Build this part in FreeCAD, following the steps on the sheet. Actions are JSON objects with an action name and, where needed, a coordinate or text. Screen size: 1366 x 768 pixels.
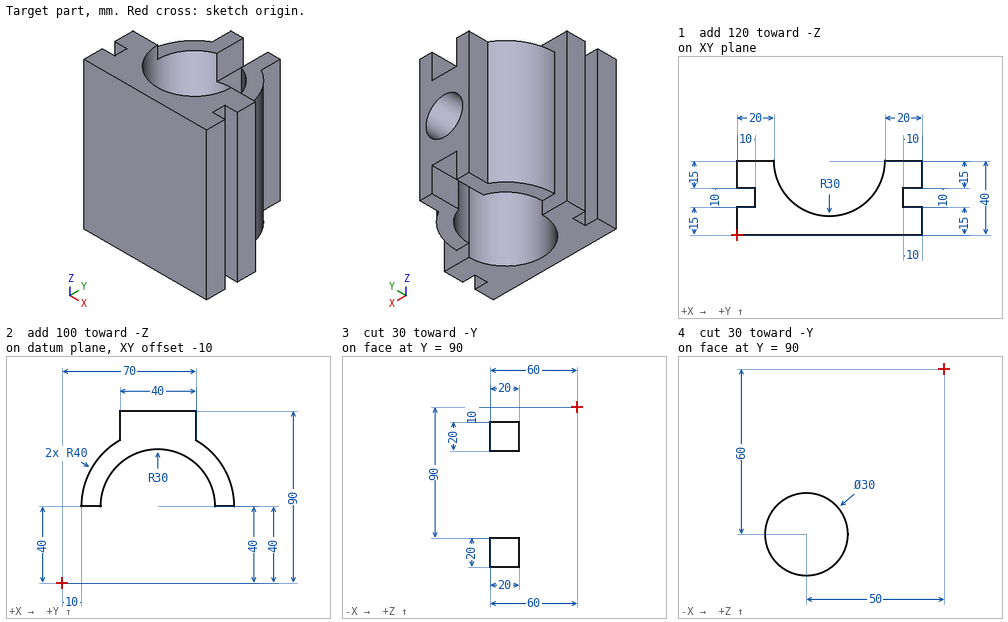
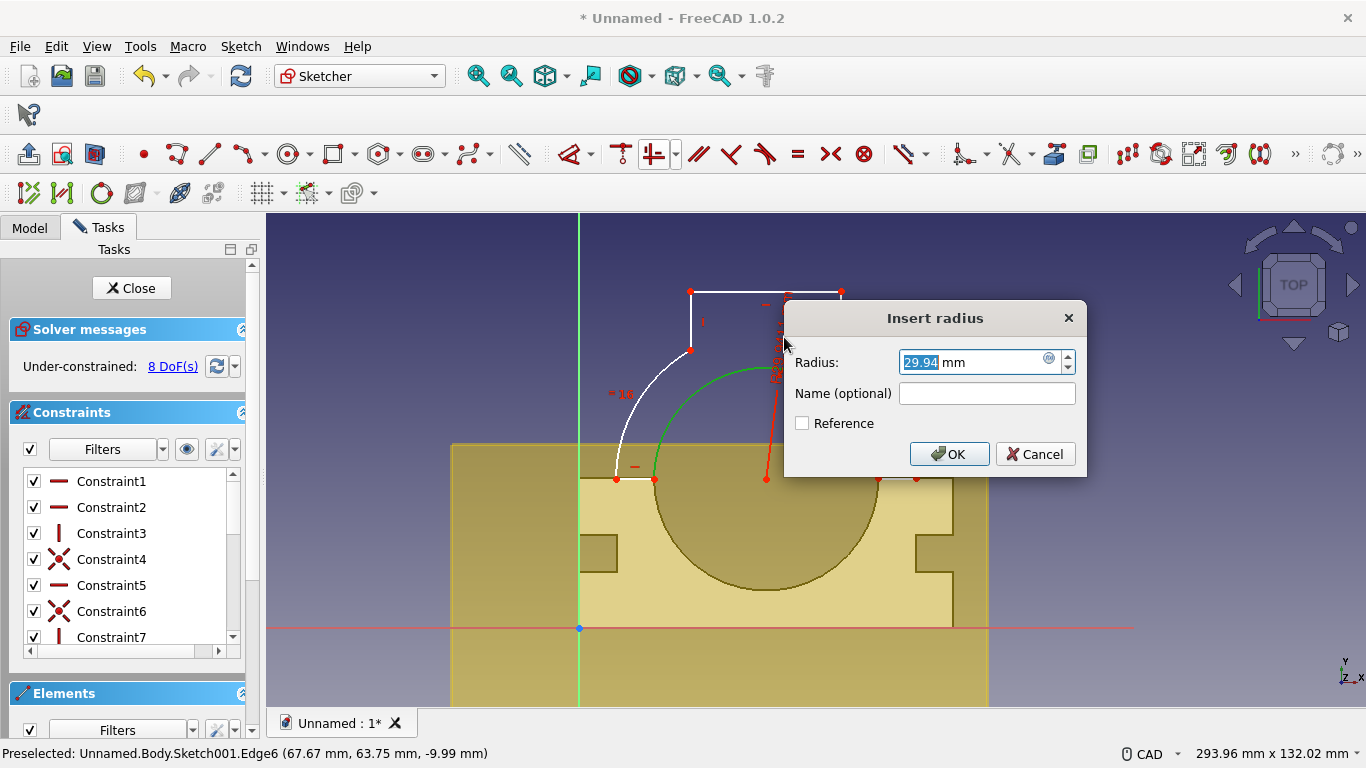
{"action": "type", "text": "30"}
{"action": "key", "text": "Return"}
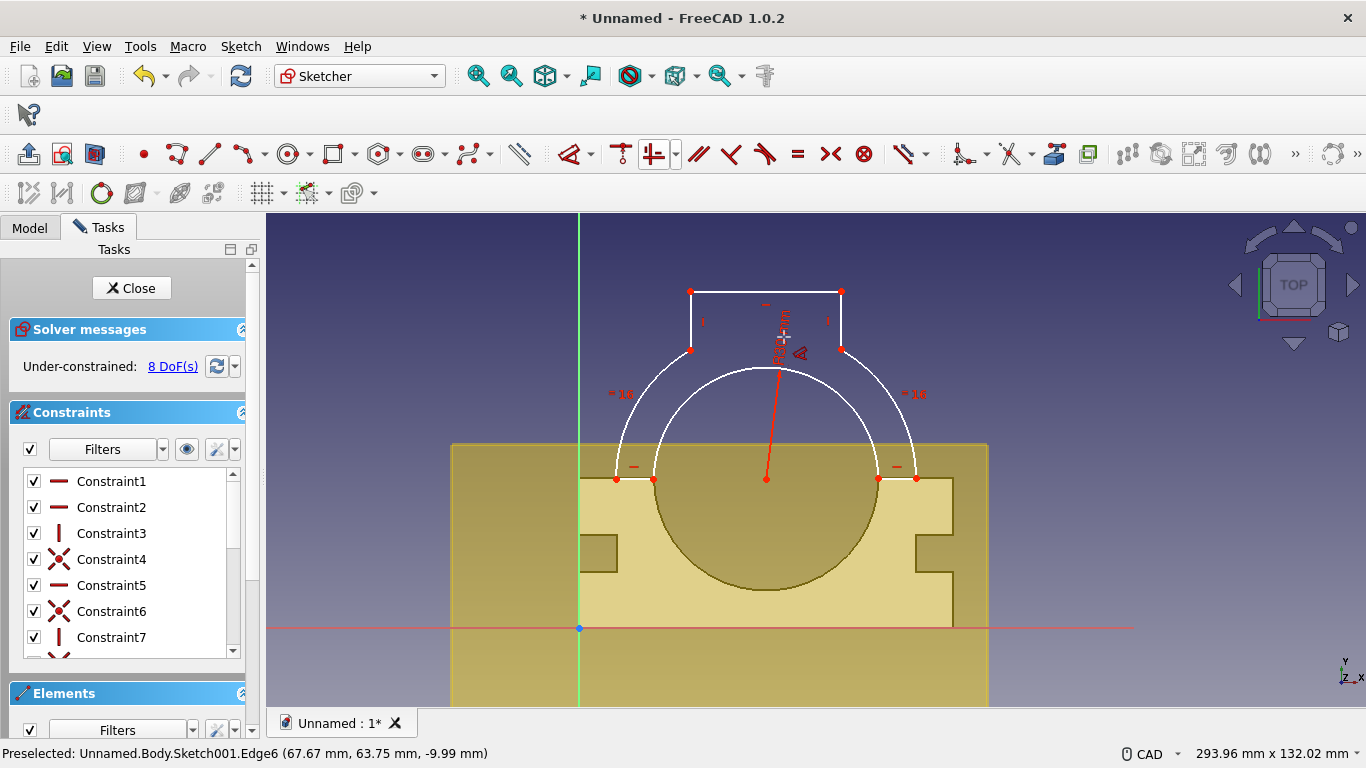
{"action": "left_click", "coordinate": [909, 433]}
{"action": "left_click", "coordinate": [939, 423]}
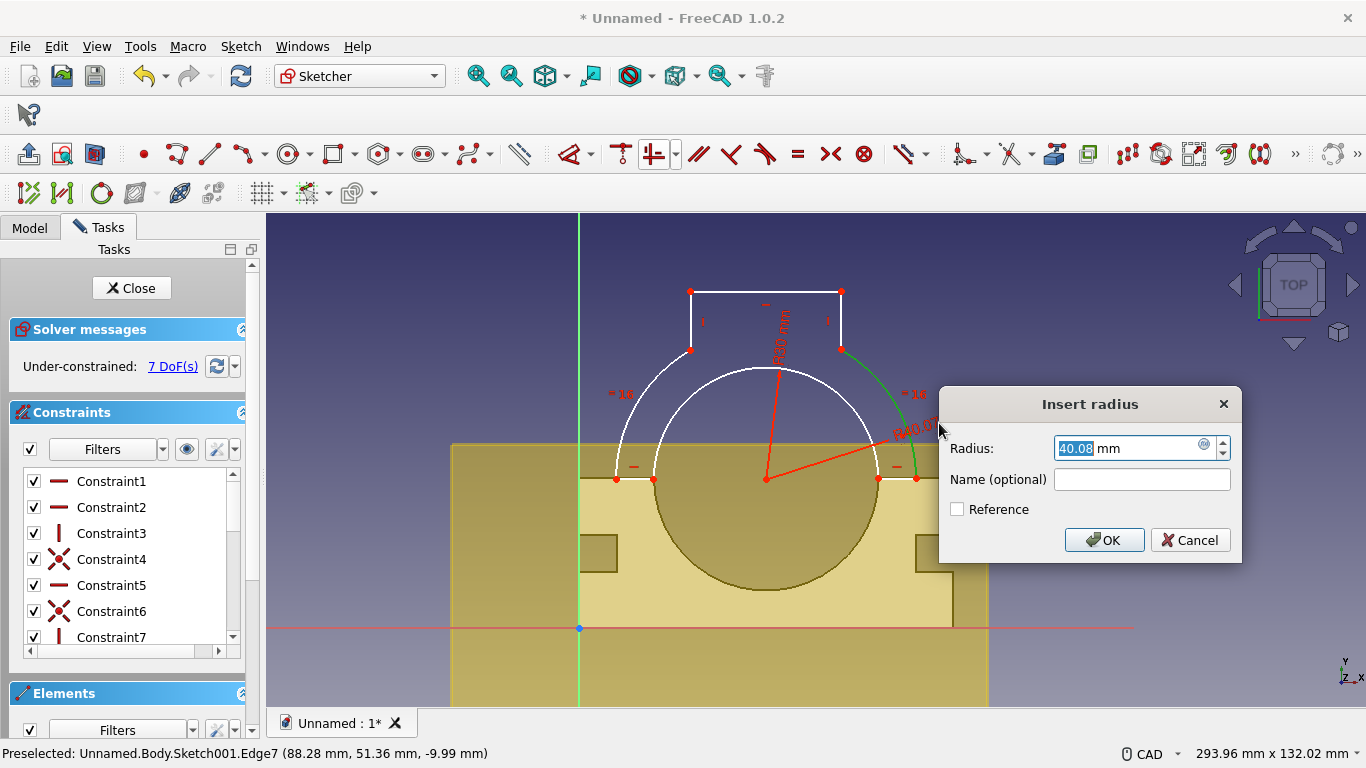
{"action": "type", "text": "40"}
{"action": "key", "text": "Return"}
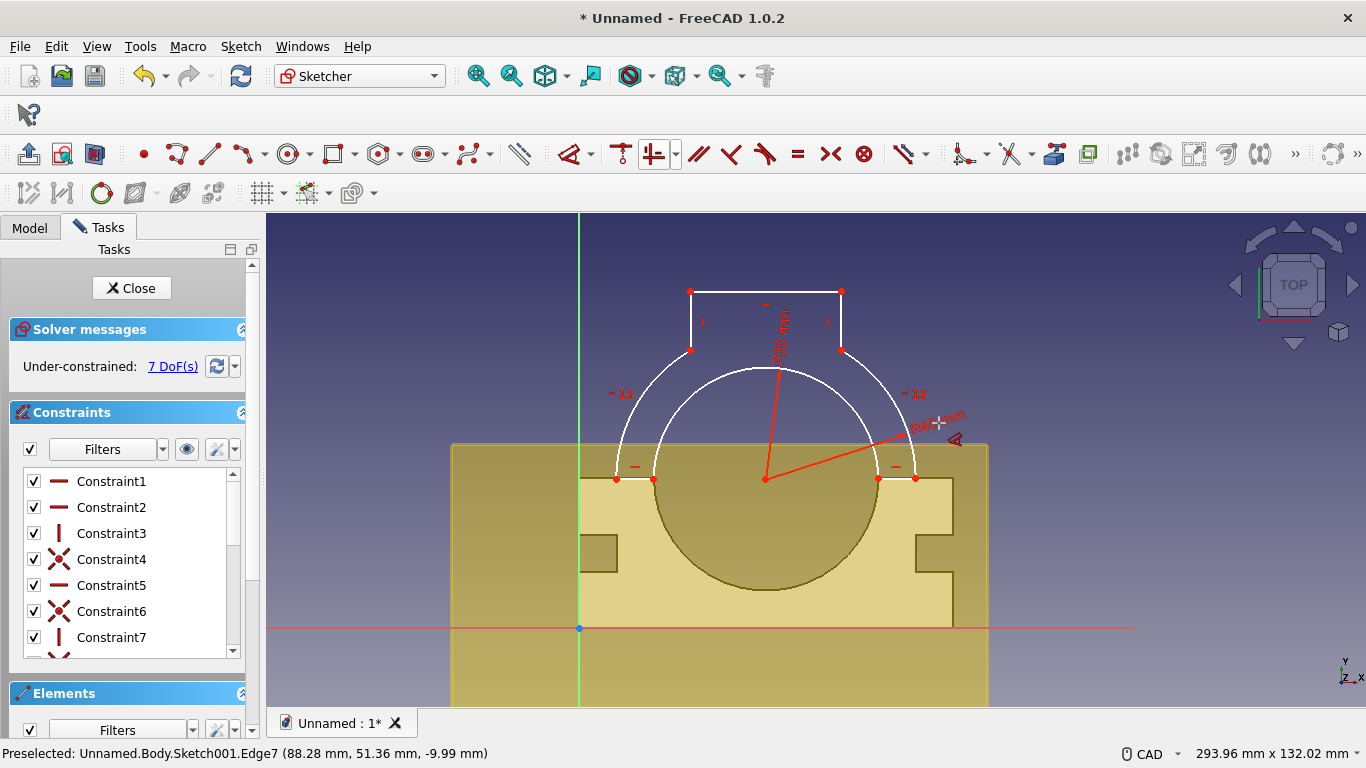
{"action": "left_click", "coordinate": [796, 292]}
{"action": "left_click", "coordinate": [766, 258]}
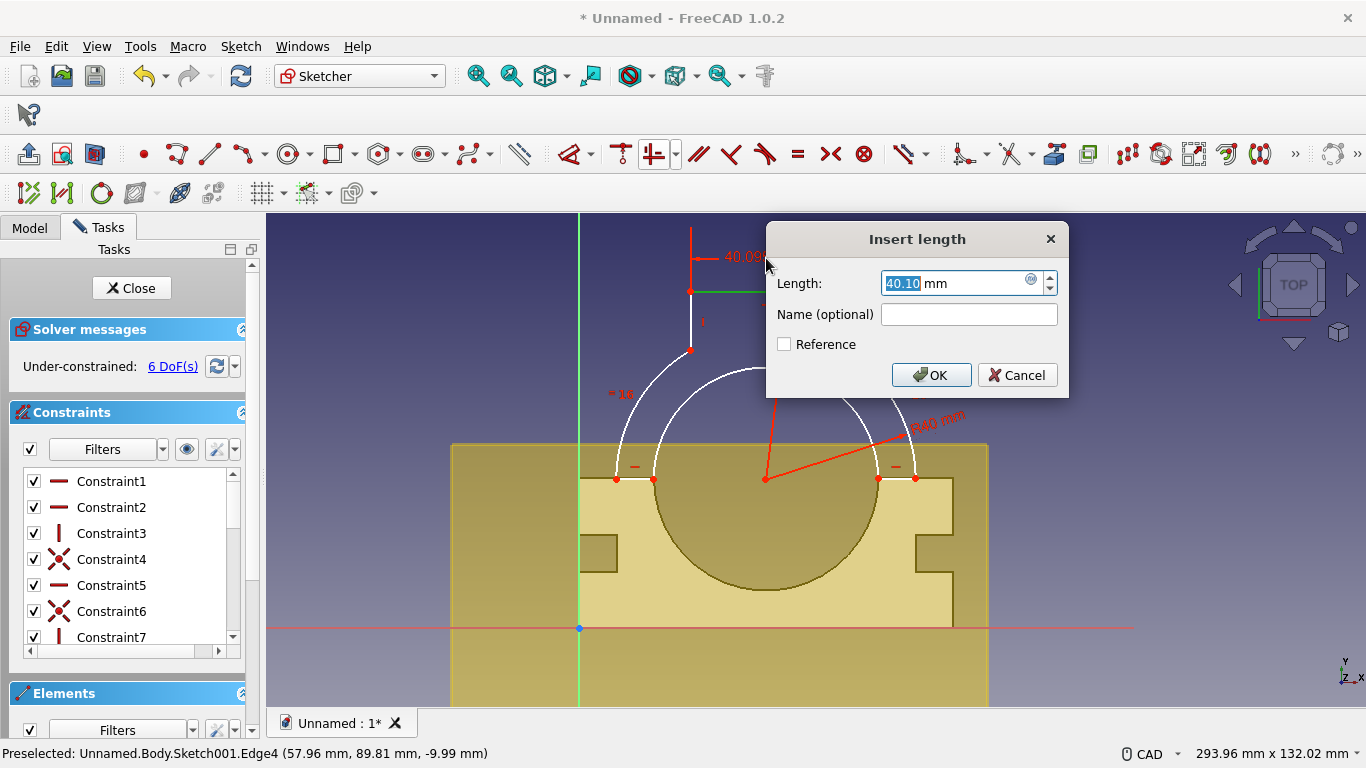
{"action": "type", "text": "40"}
{"action": "key", "text": "Return"}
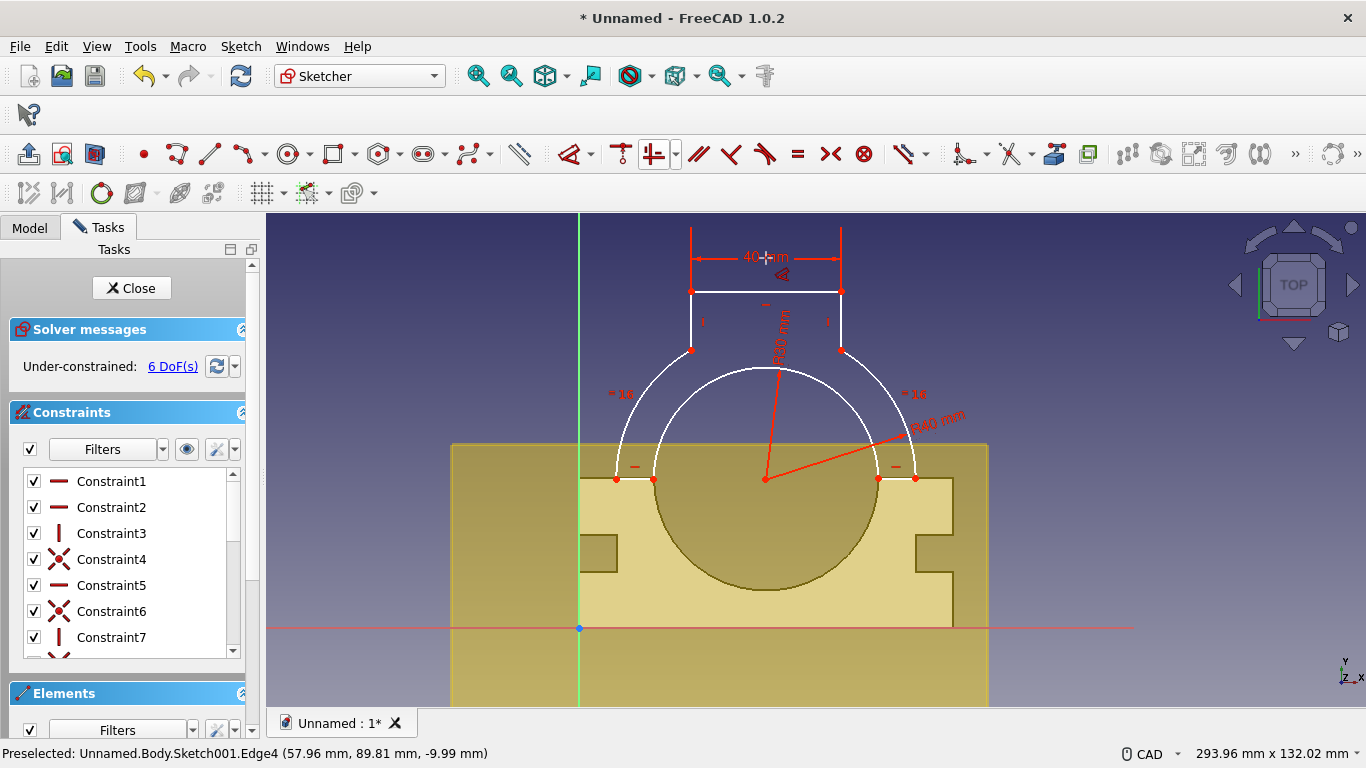
{"action": "left_click", "coordinate": [616, 479]}
{"action": "left_click", "coordinate": [598, 662]}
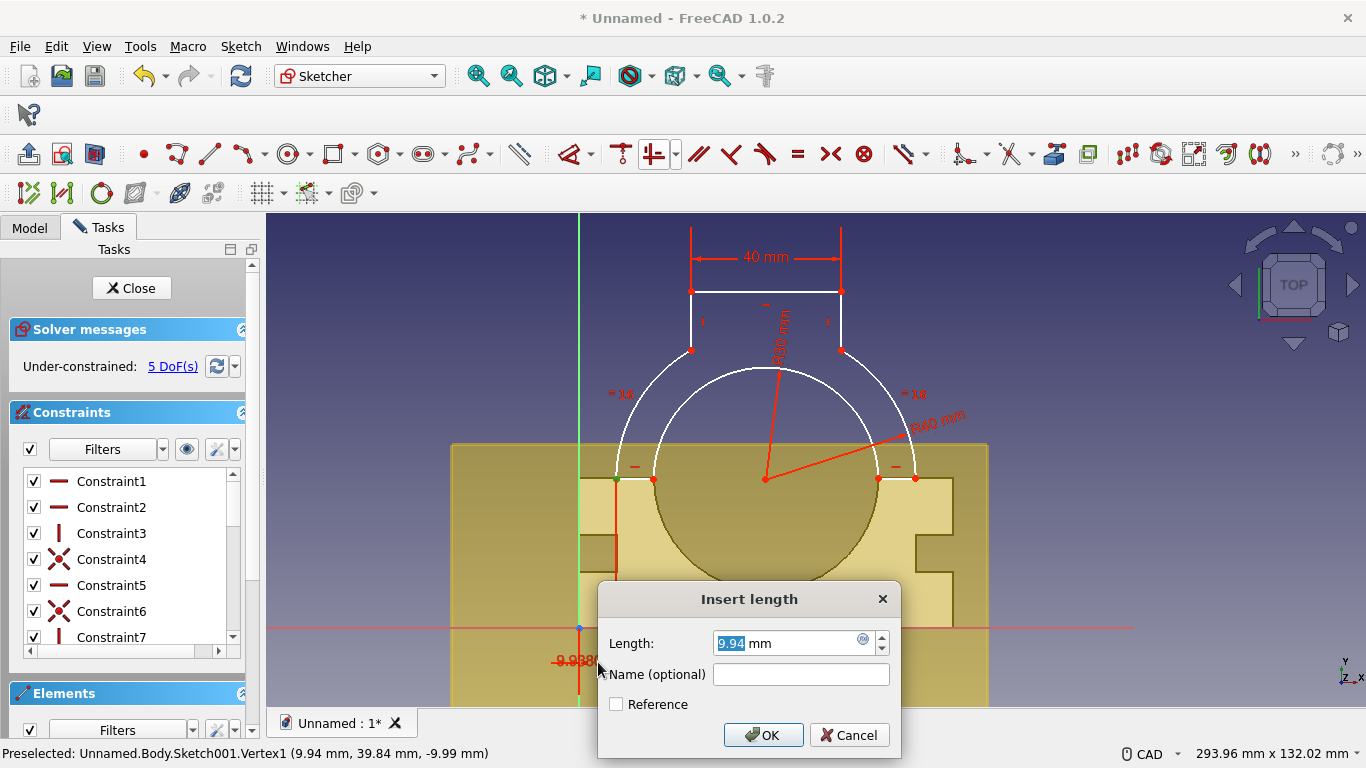
{"action": "type", "text": "10"}
{"action": "key", "text": "Return"}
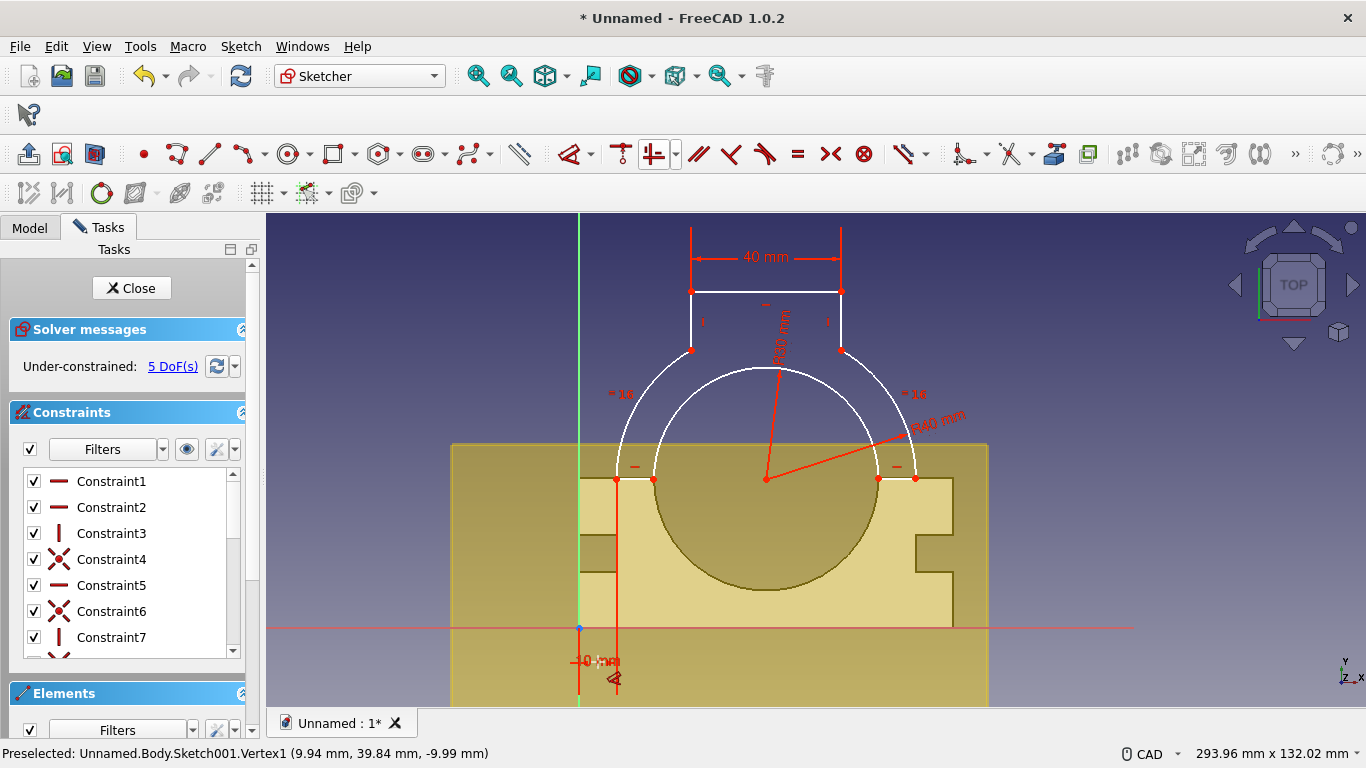
{"action": "left_click", "coordinate": [617, 479]}
{"action": "left_click", "coordinate": [545, 554]}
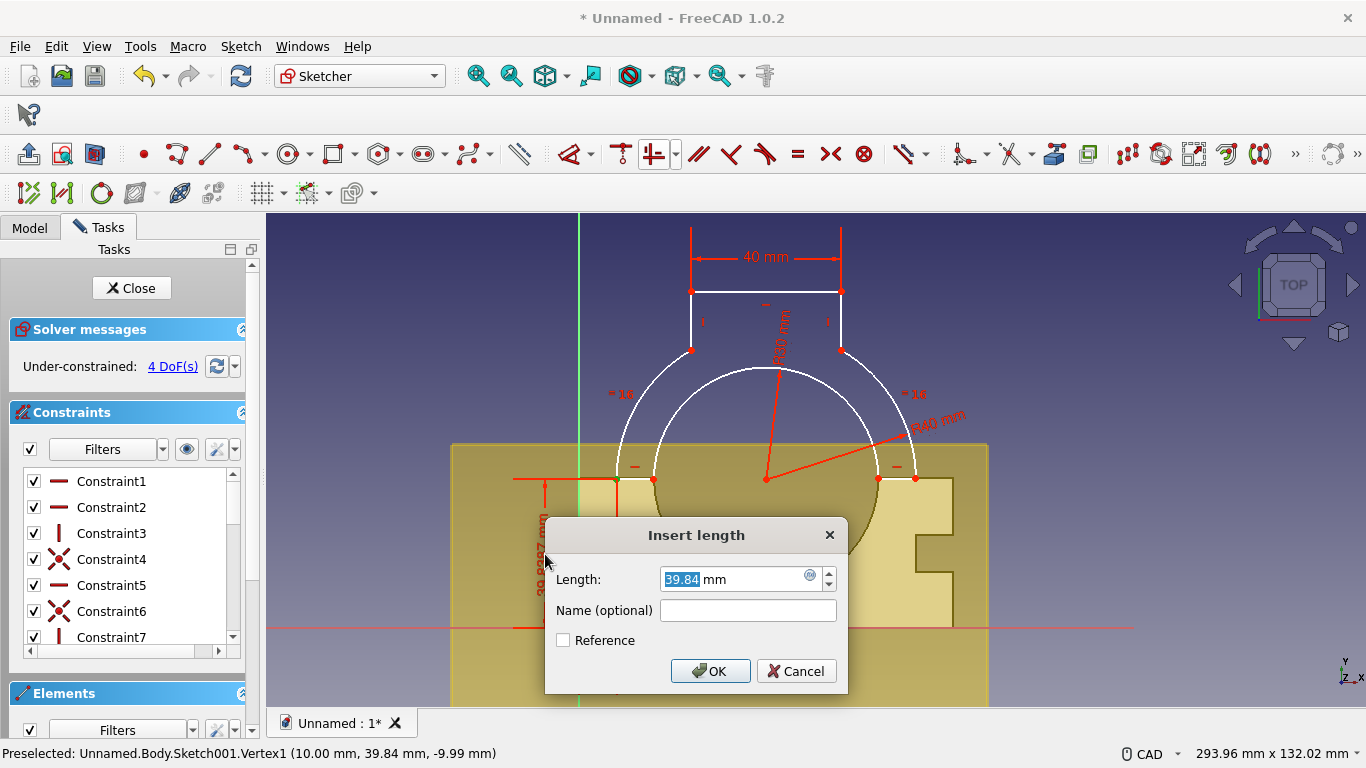
{"action": "type", "text": "40"}
{"action": "key", "text": "Return"}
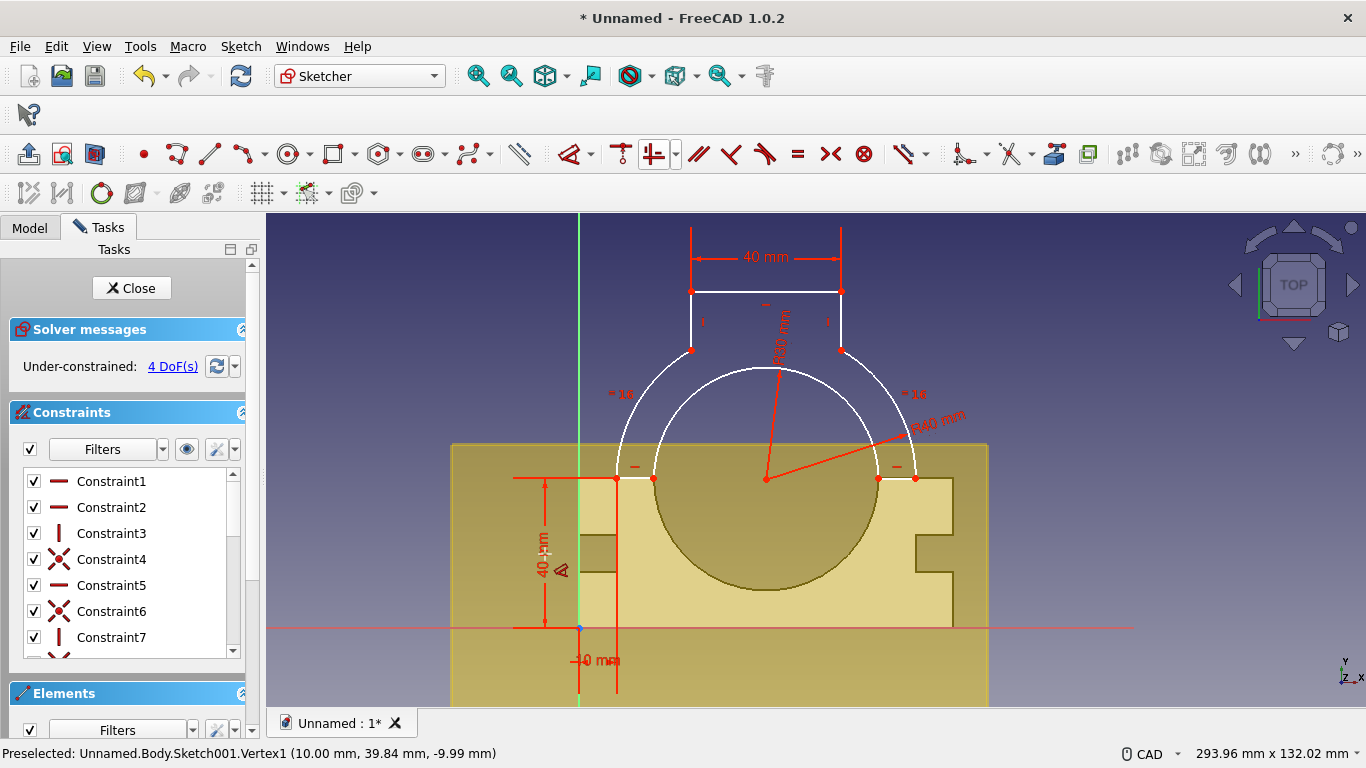
{"action": "left_click", "coordinate": [878, 479]}
{"action": "left_click", "coordinate": [545, 519]}